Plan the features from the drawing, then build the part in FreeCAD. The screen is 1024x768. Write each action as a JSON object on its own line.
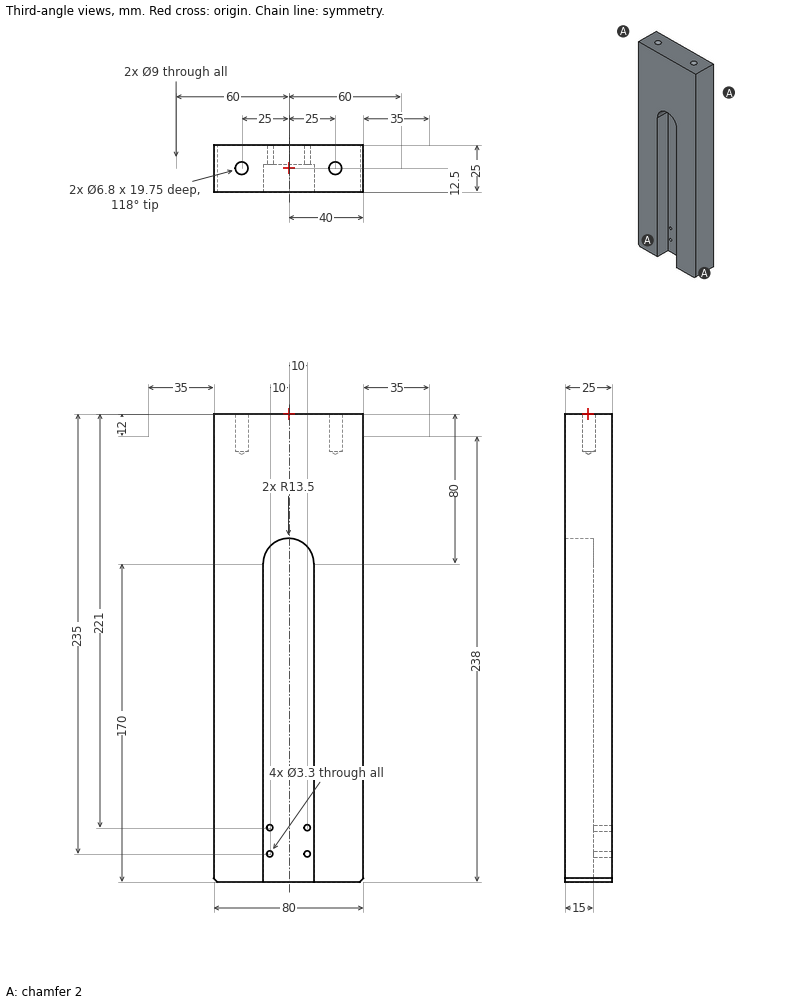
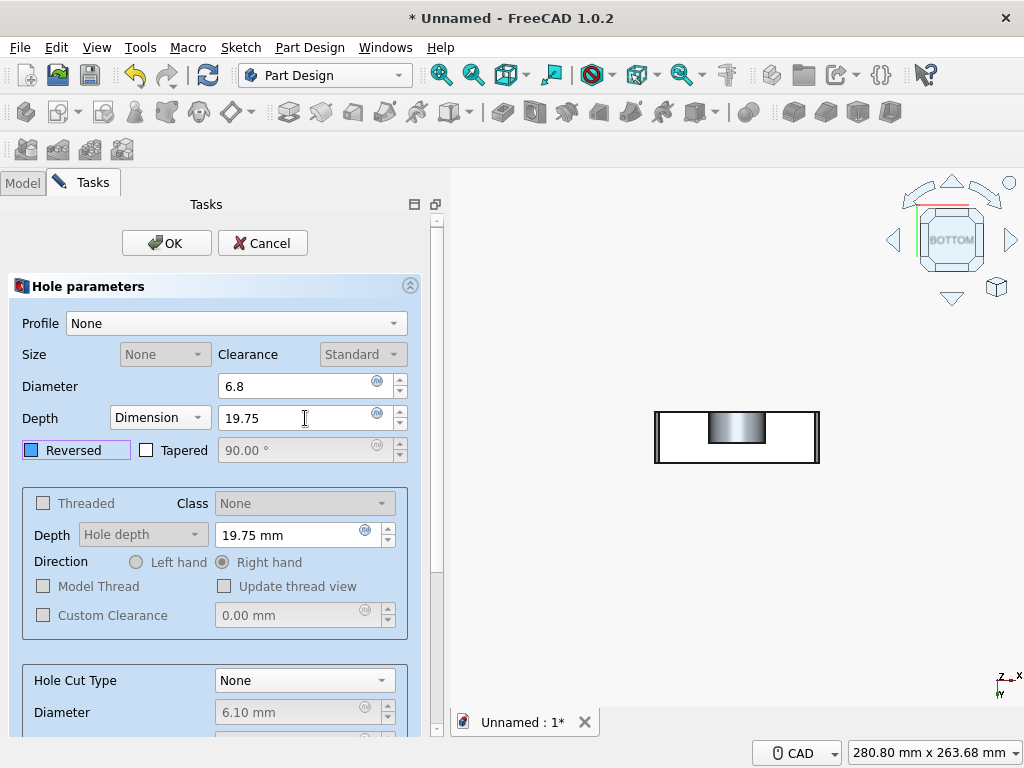
{"action": "left_click", "coordinate": [167, 243]}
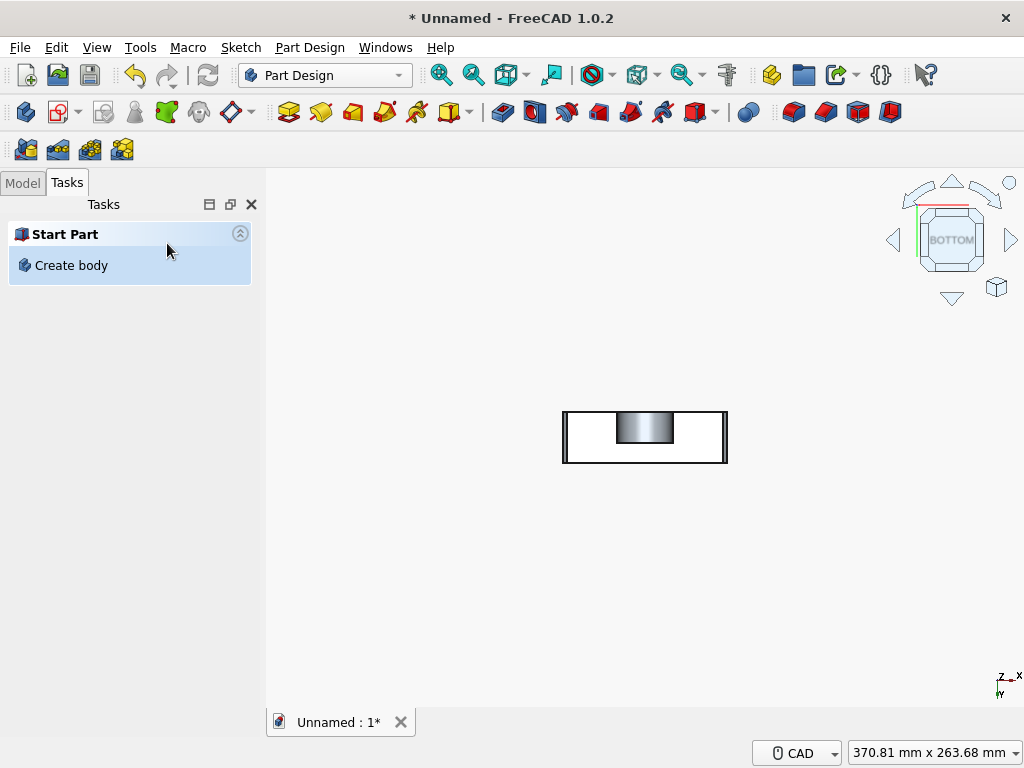
{"action": "key", "text": "0"}